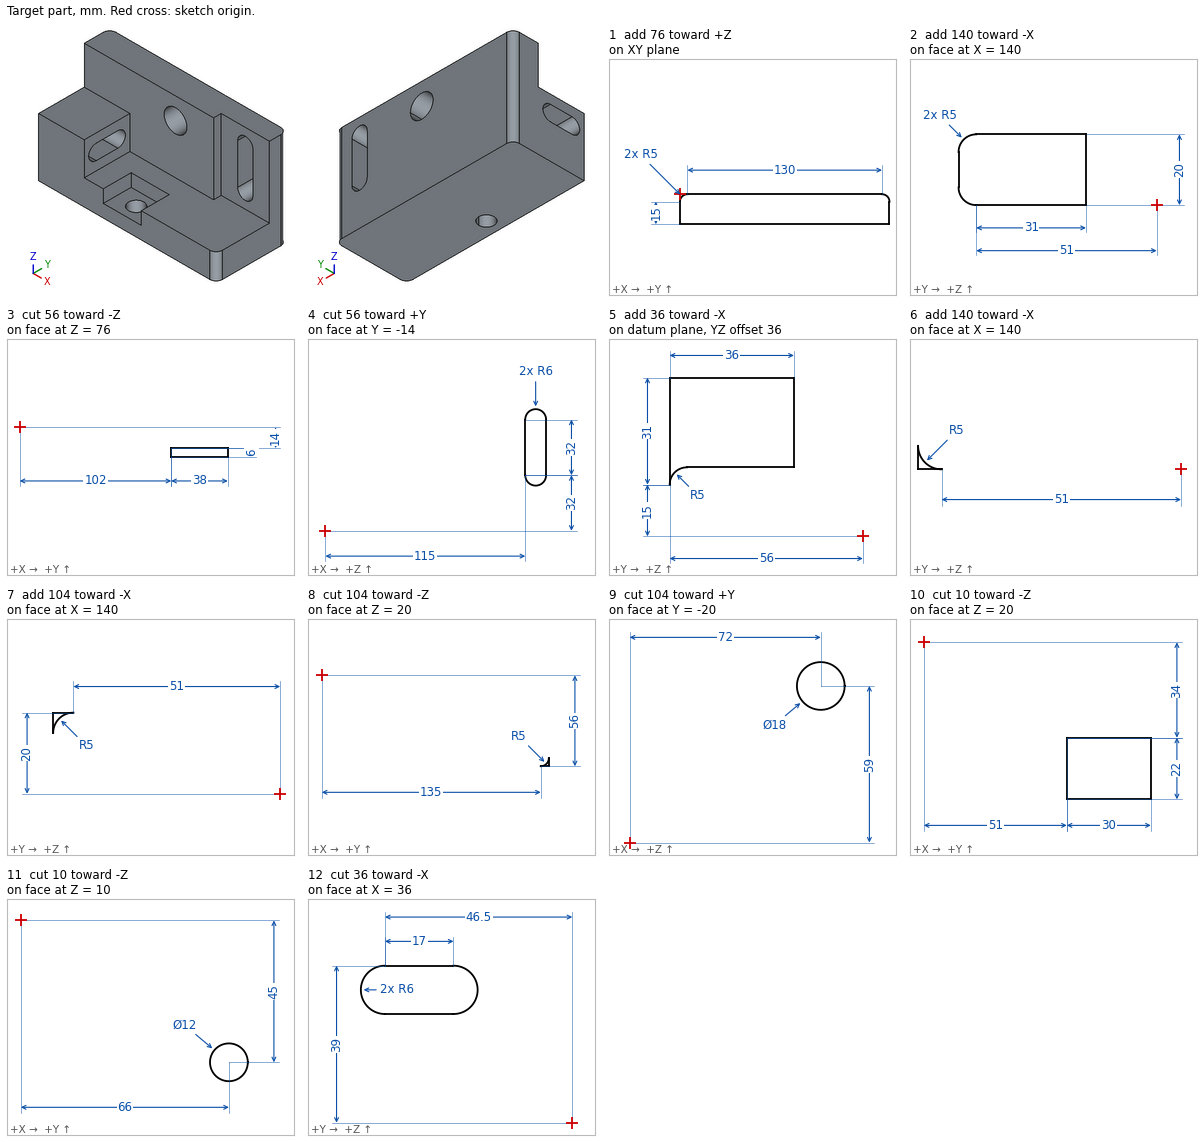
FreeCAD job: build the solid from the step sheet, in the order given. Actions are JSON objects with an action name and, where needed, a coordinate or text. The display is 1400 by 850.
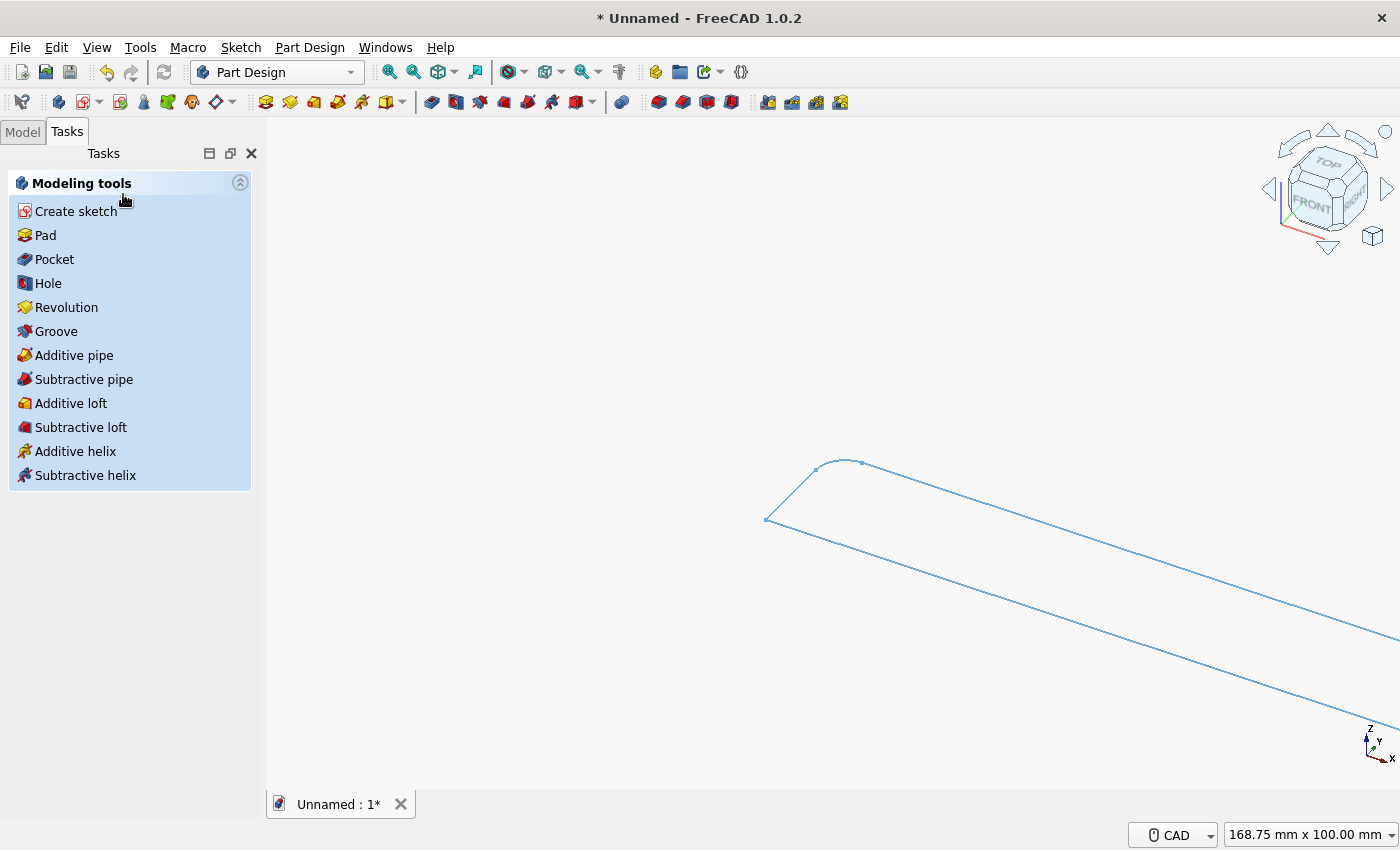
{"action": "left_click", "coordinate": [266, 102]}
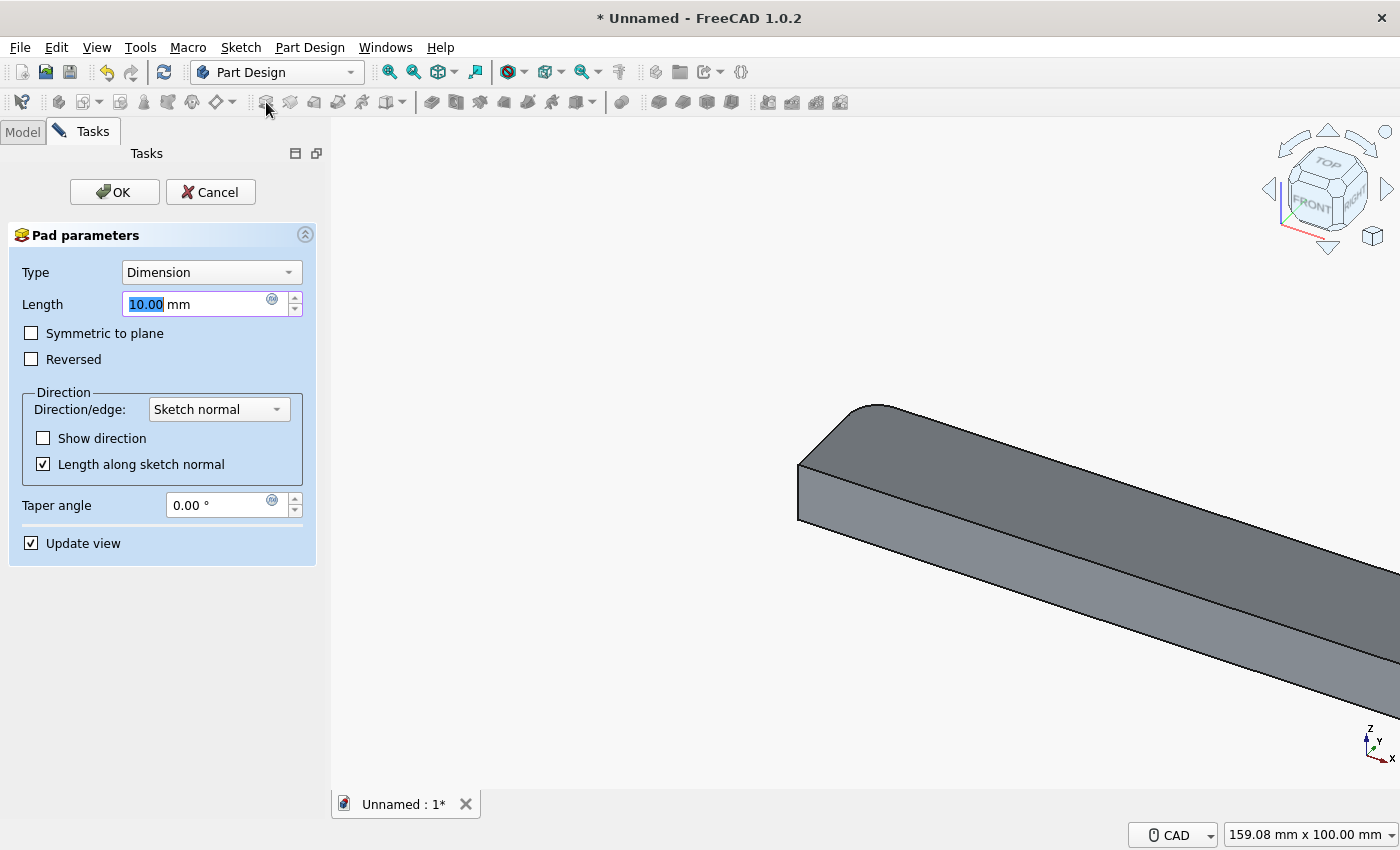
{"action": "type", "text": "76"}
{"action": "key", "text": "Tab"}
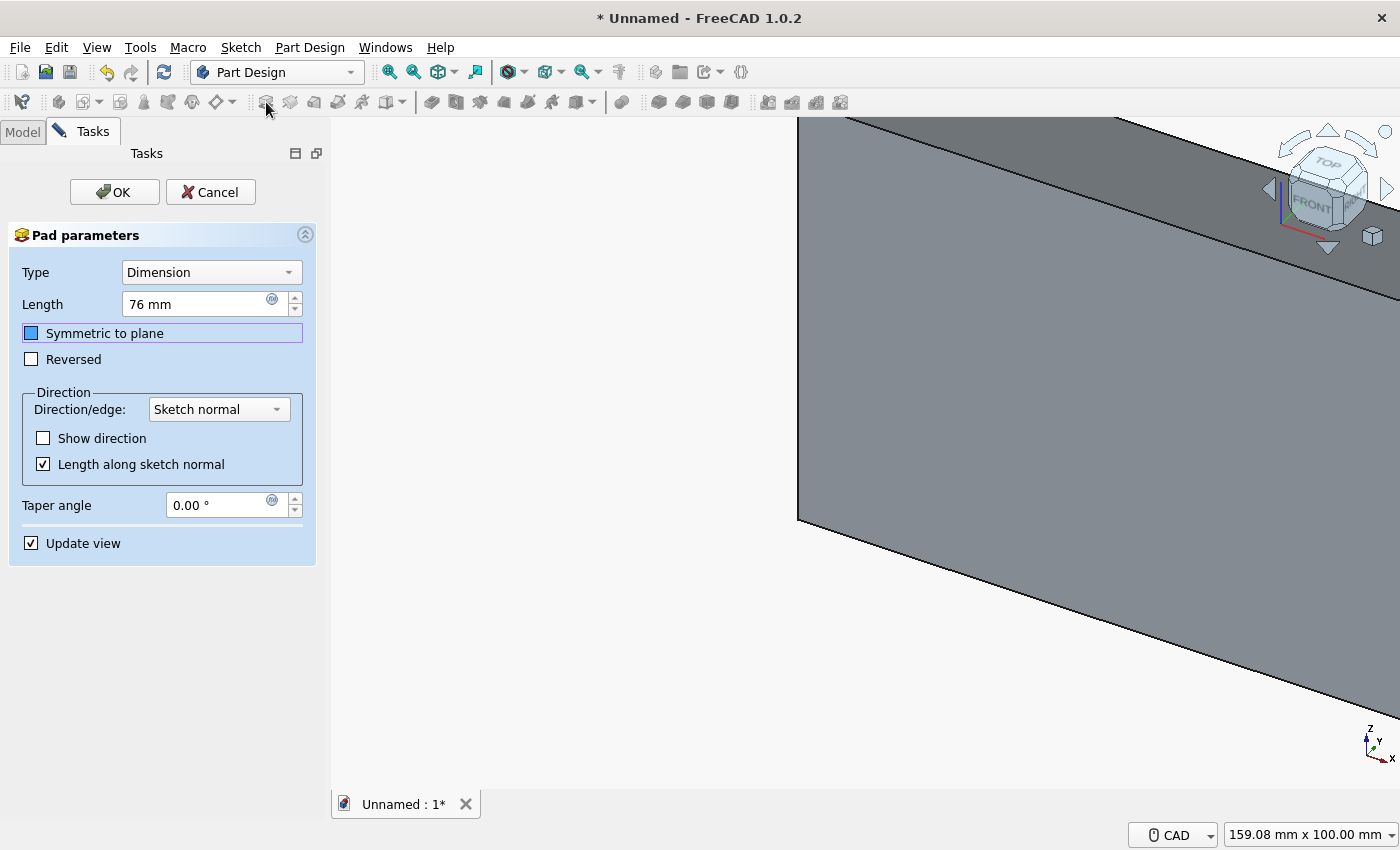
{"action": "left_click", "coordinate": [115, 192]}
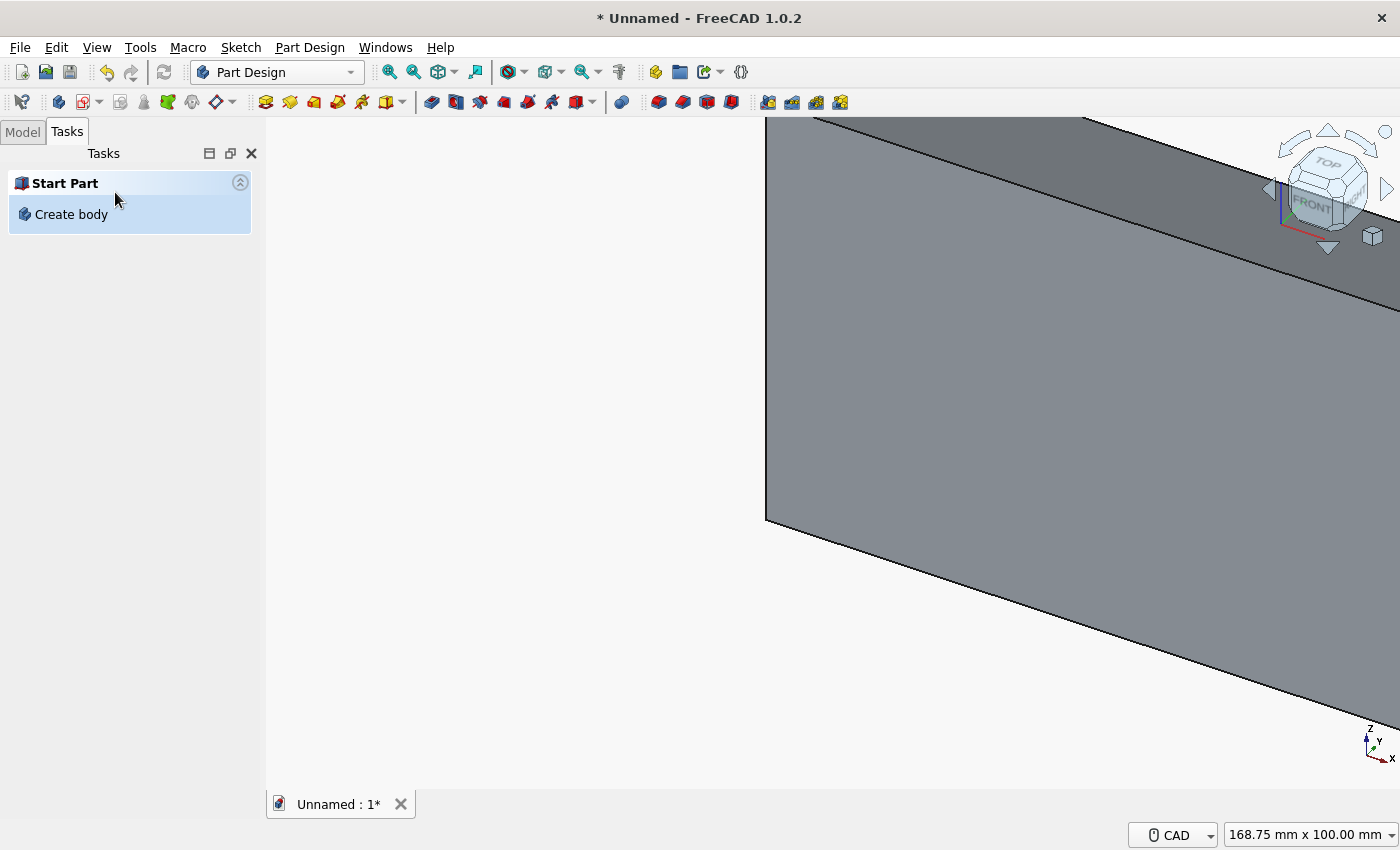
{"action": "key", "text": "v f"}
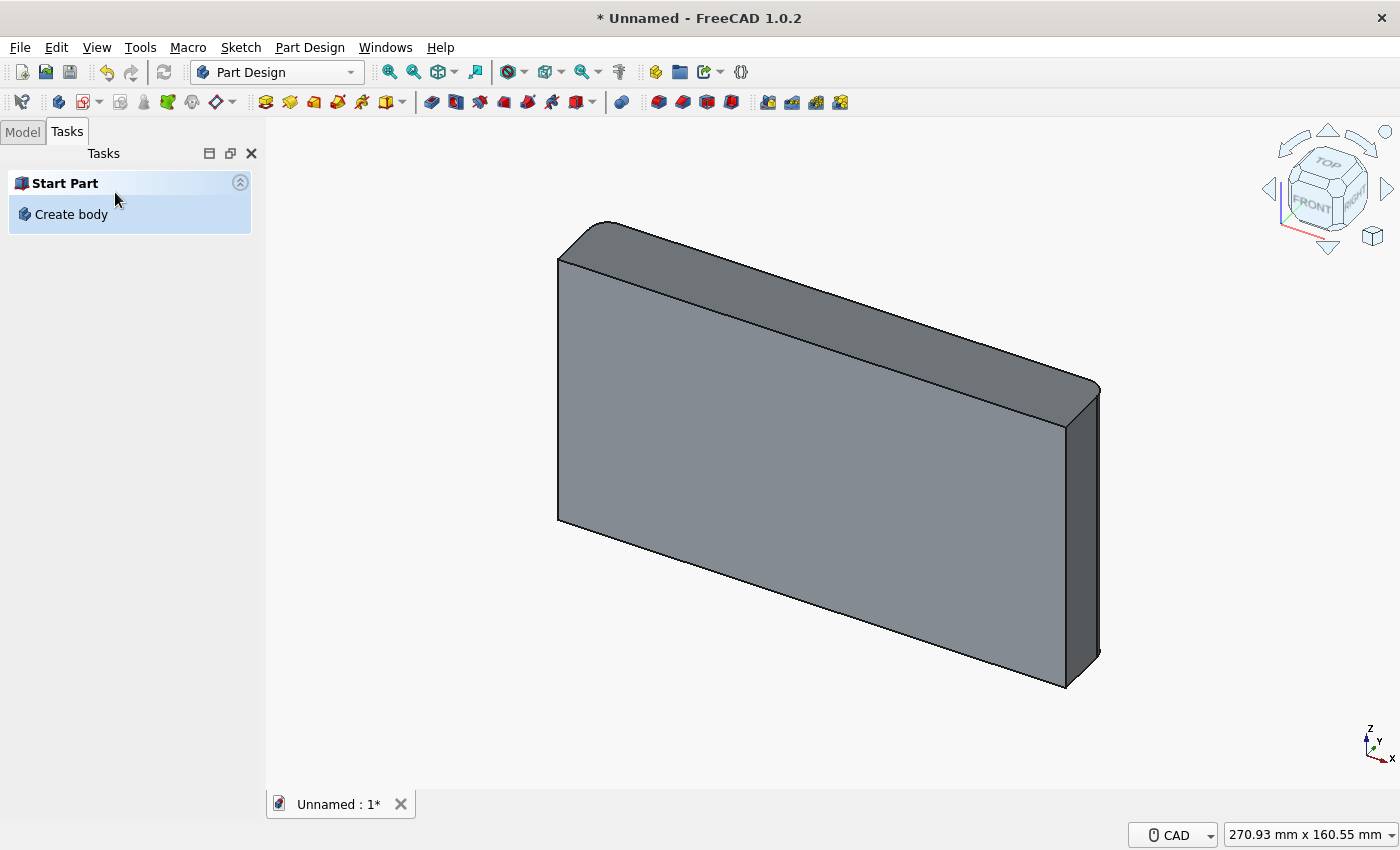
{"action": "left_click", "coordinate": [1082, 467]}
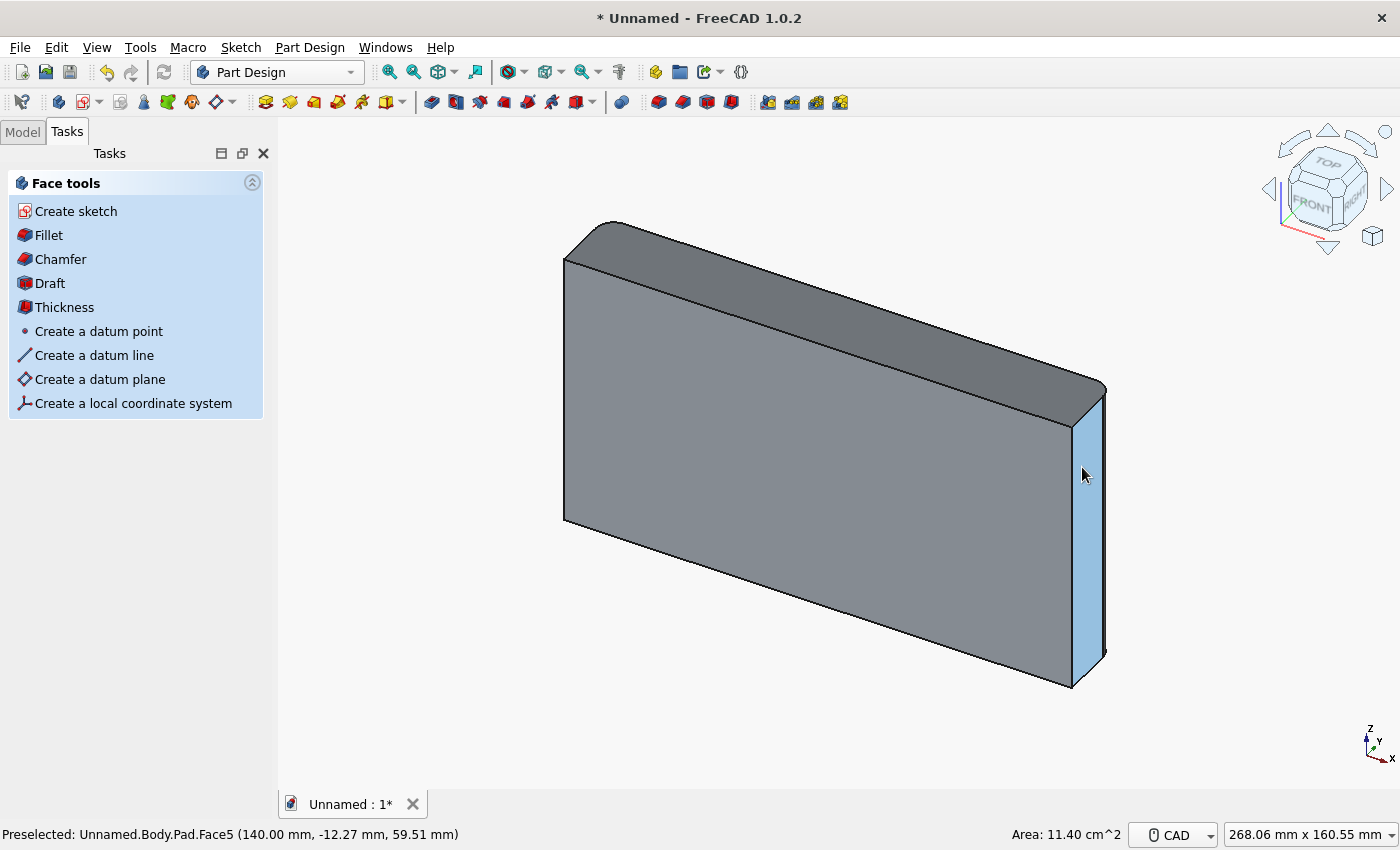
{"action": "left_click", "coordinate": [84, 102]}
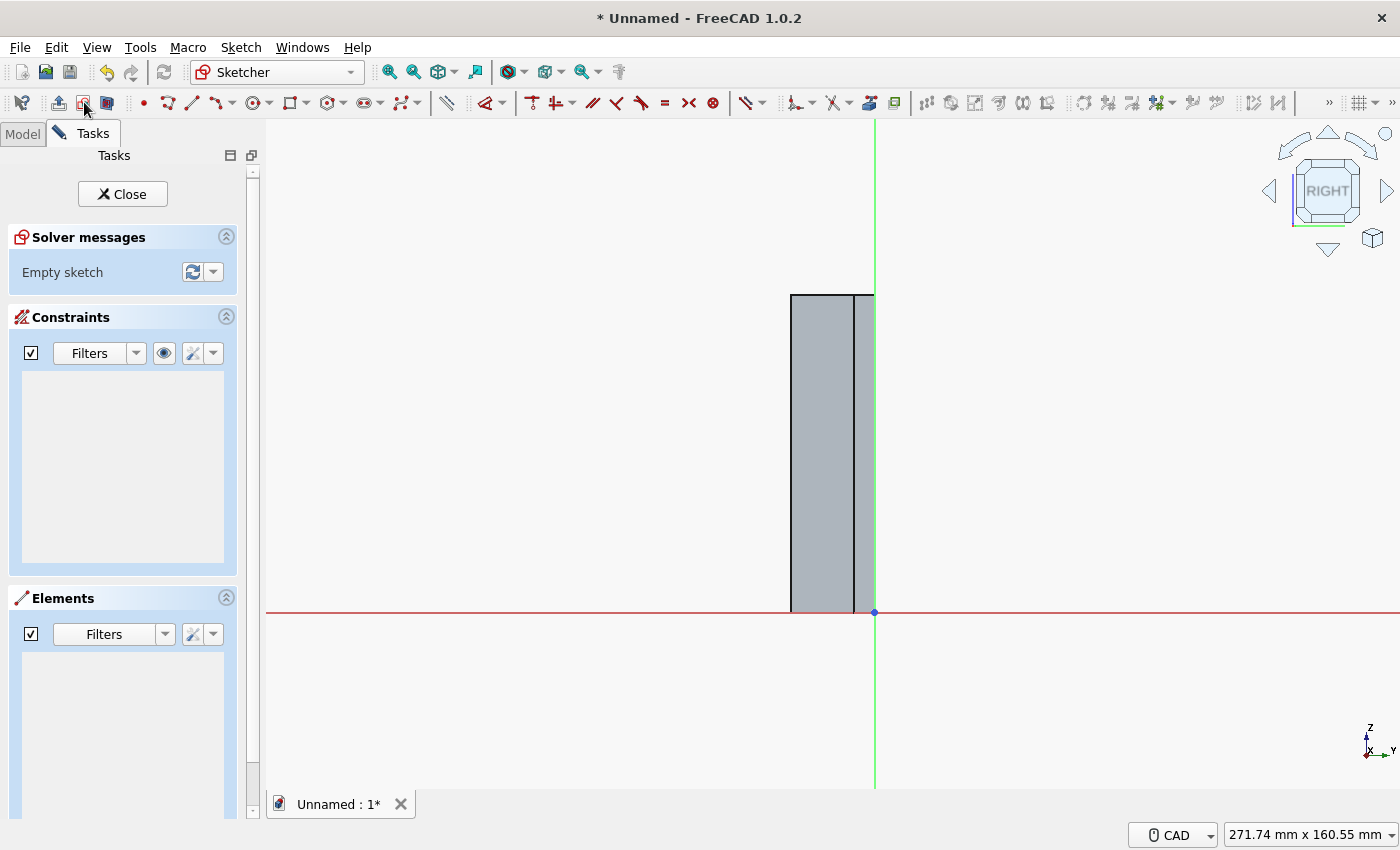
{"action": "scroll", "coordinate": [754, 639], "scroll_direction": "up", "scroll_amount": 5}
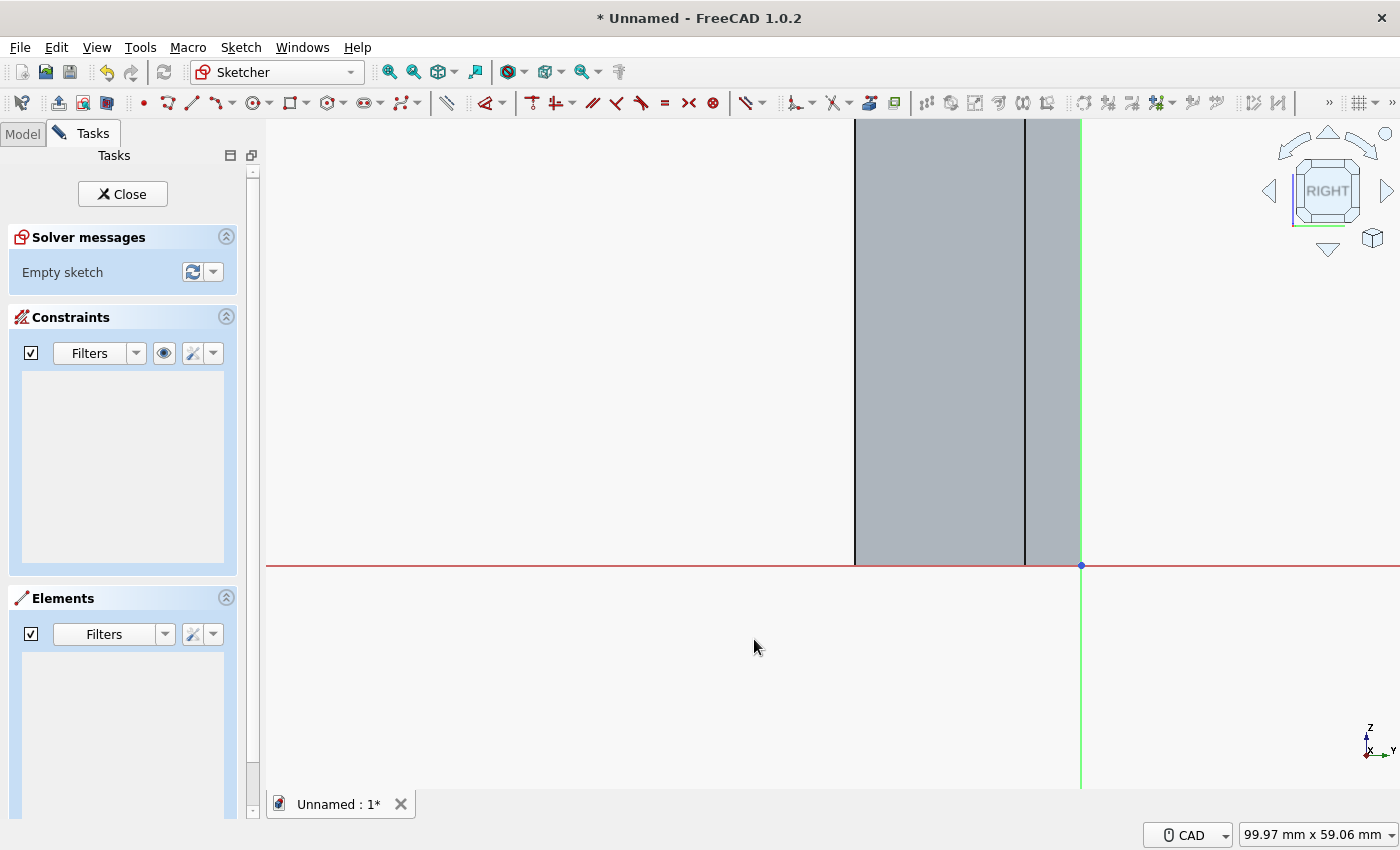
{"action": "left_click", "coordinate": [168, 104]}